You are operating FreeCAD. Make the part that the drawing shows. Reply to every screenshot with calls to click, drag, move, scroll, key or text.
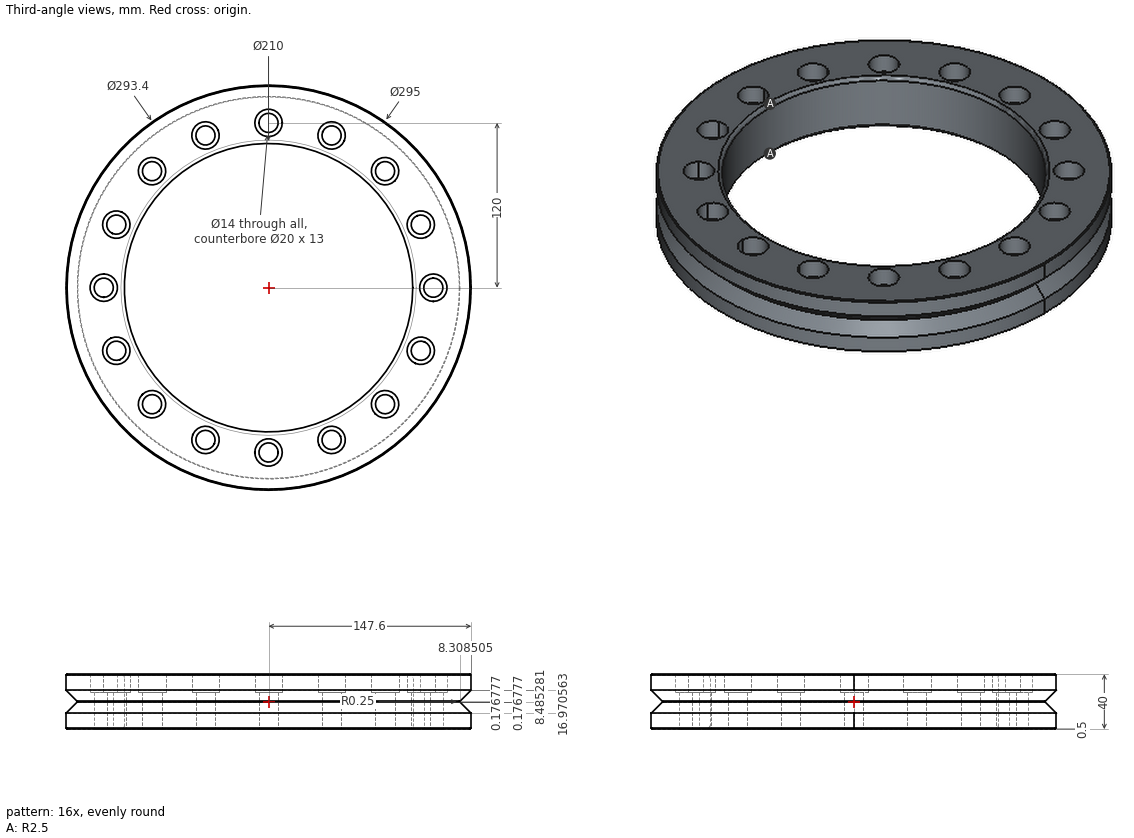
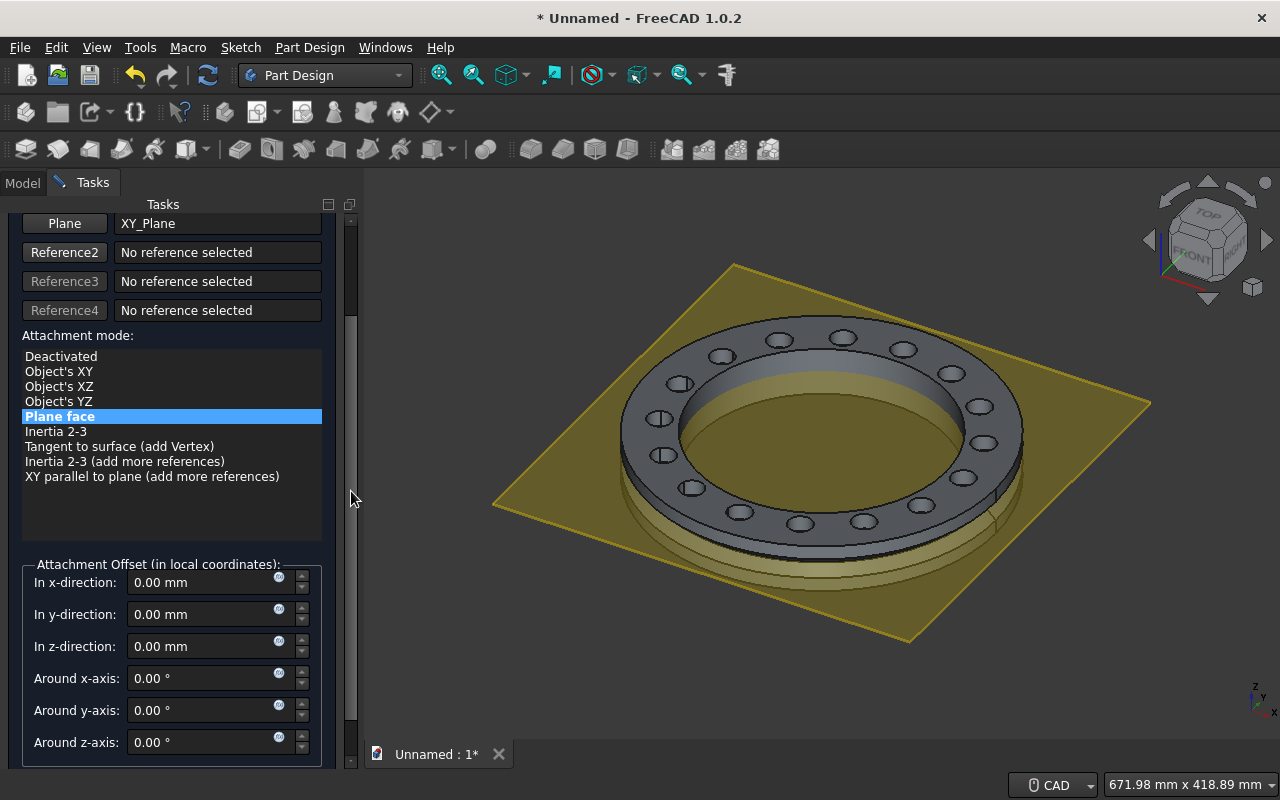
triple_click(210, 646)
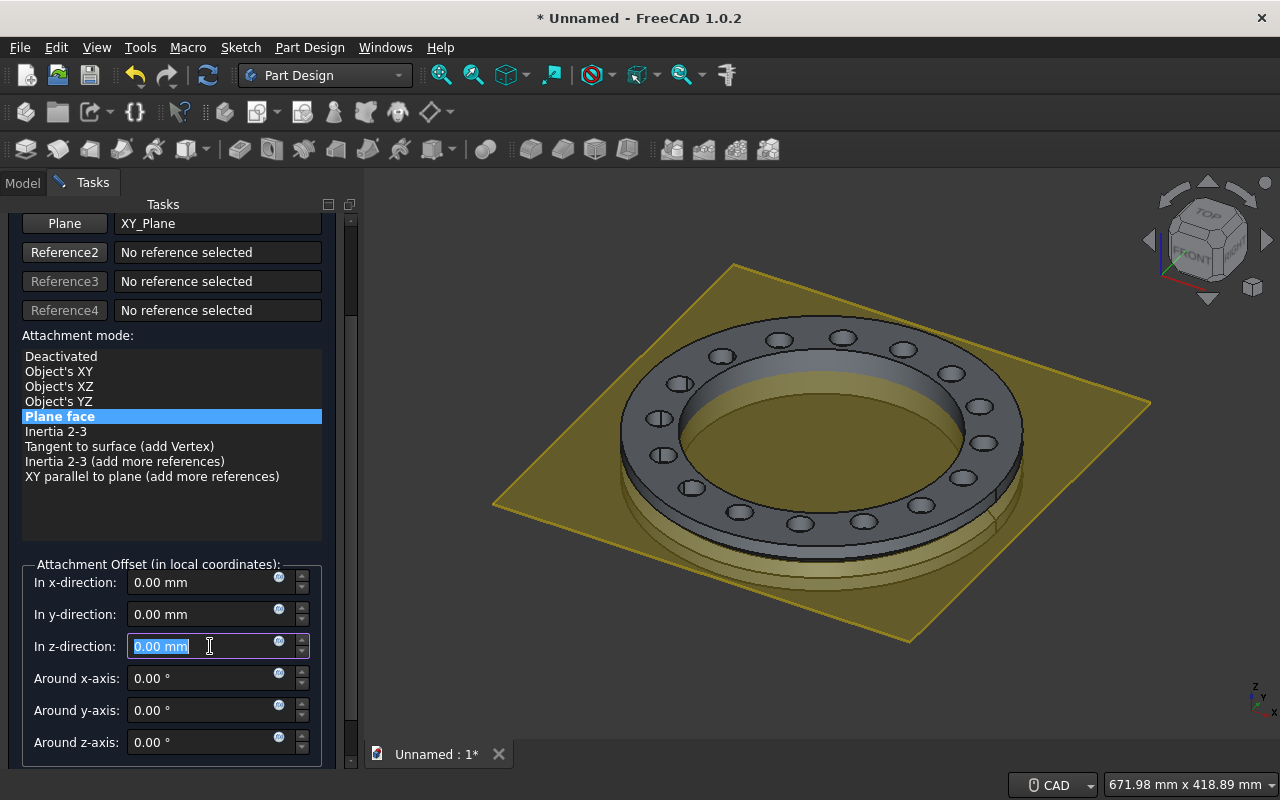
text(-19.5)
key(Tab)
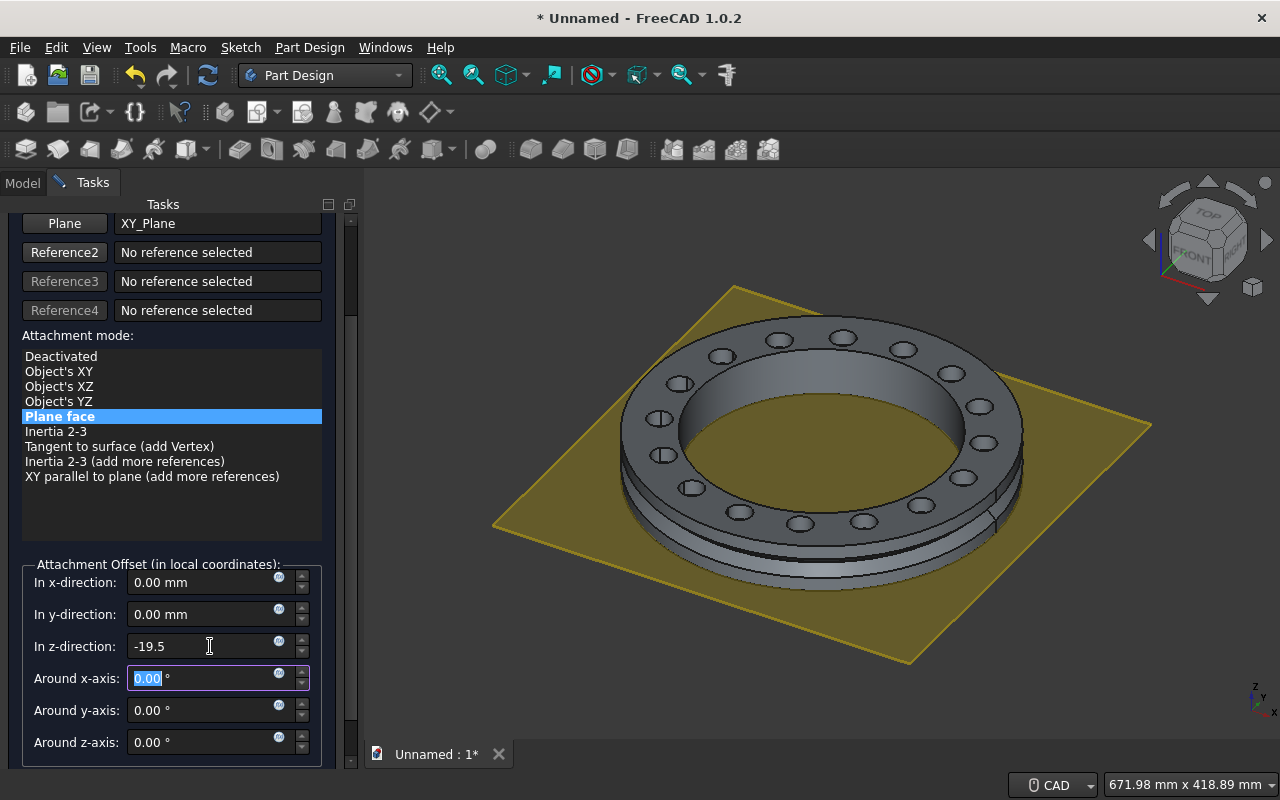
scroll(351, 491, up, 3)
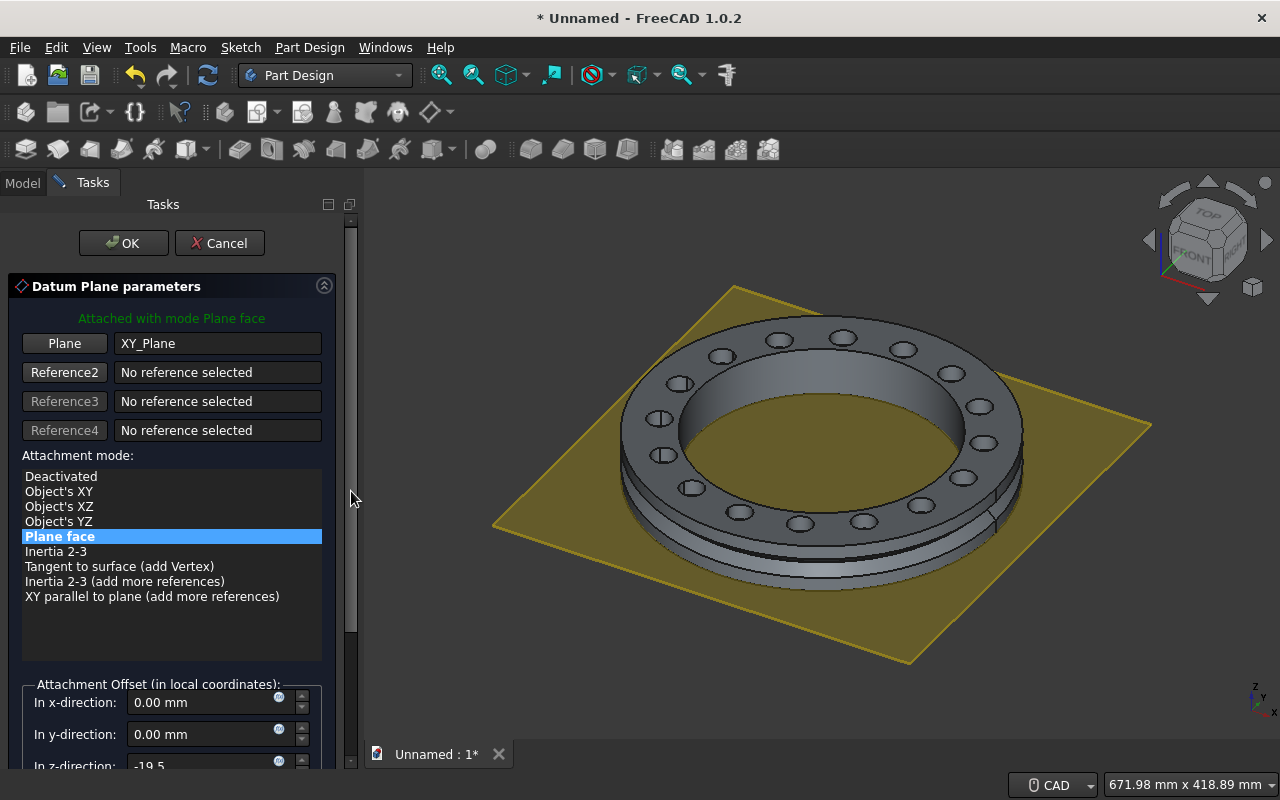
click(124, 243)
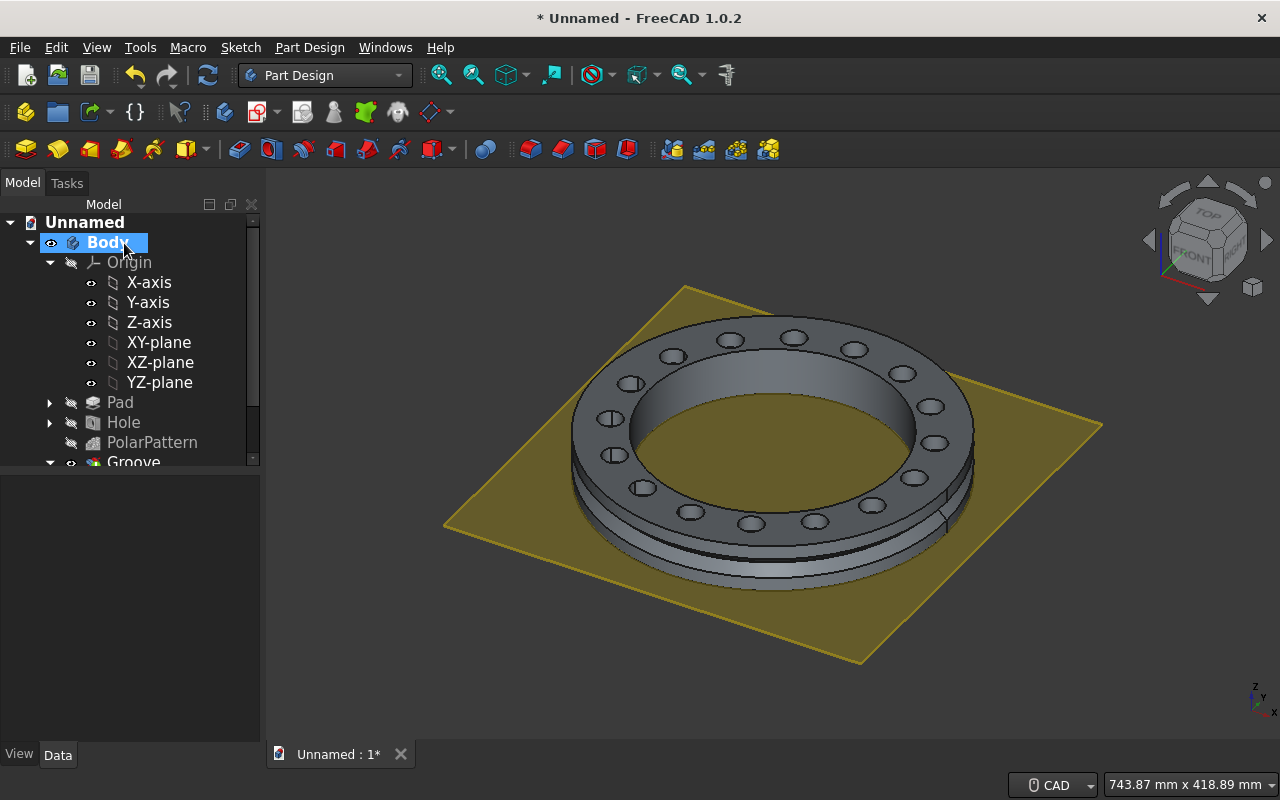
scroll(100, 338, down, 3)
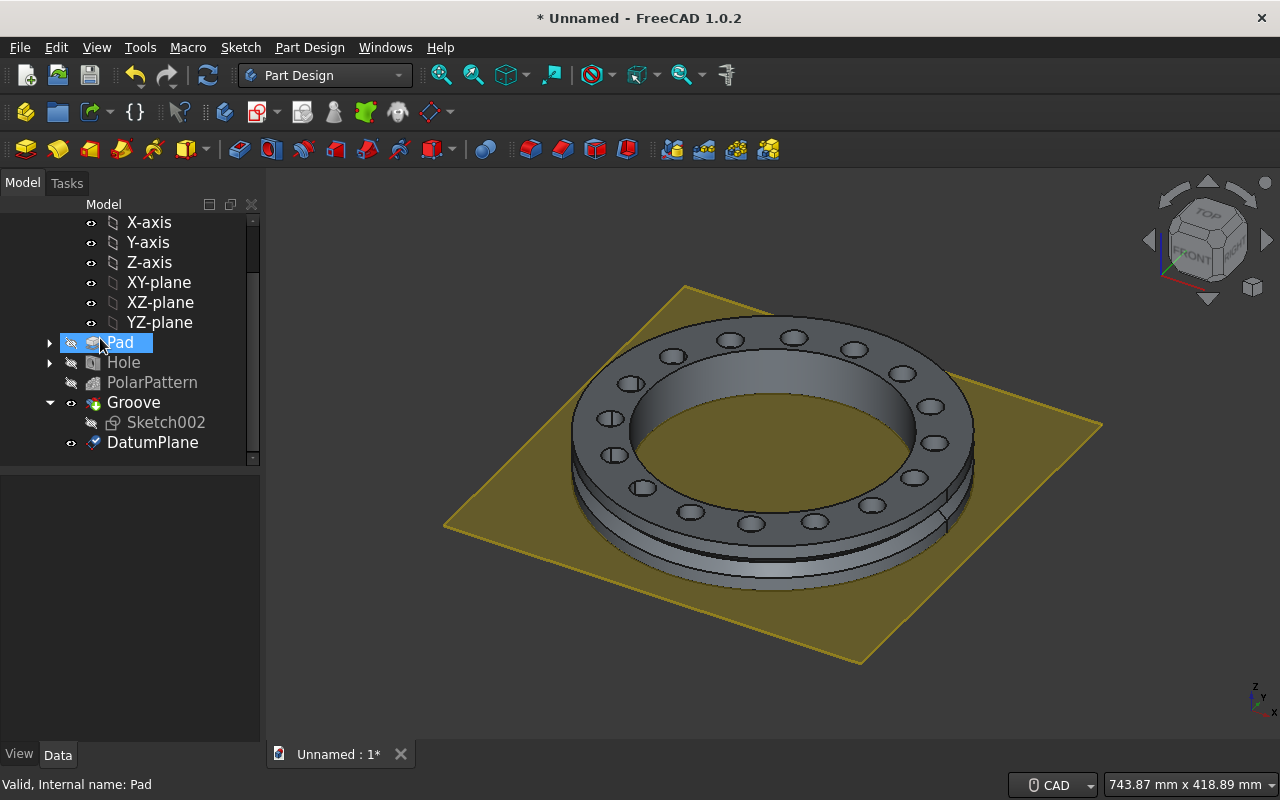
click(116, 443)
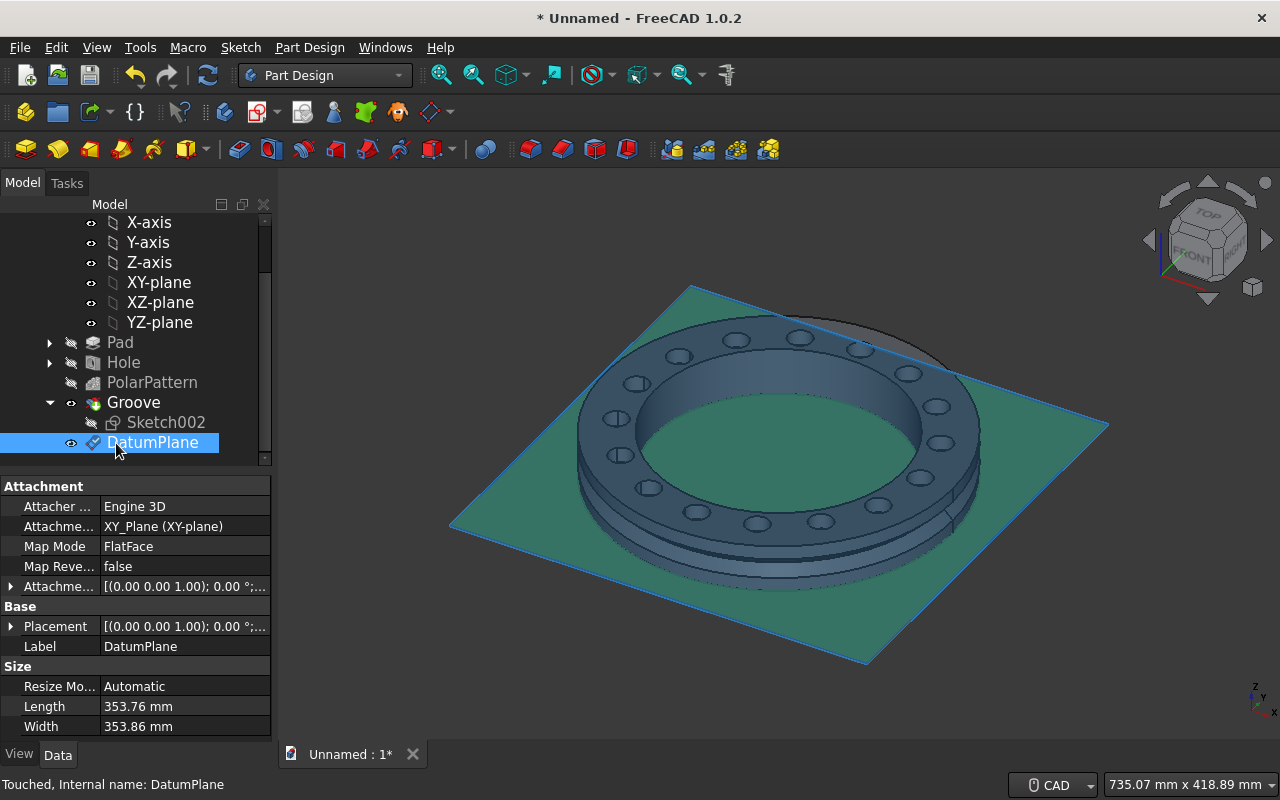
click(258, 112)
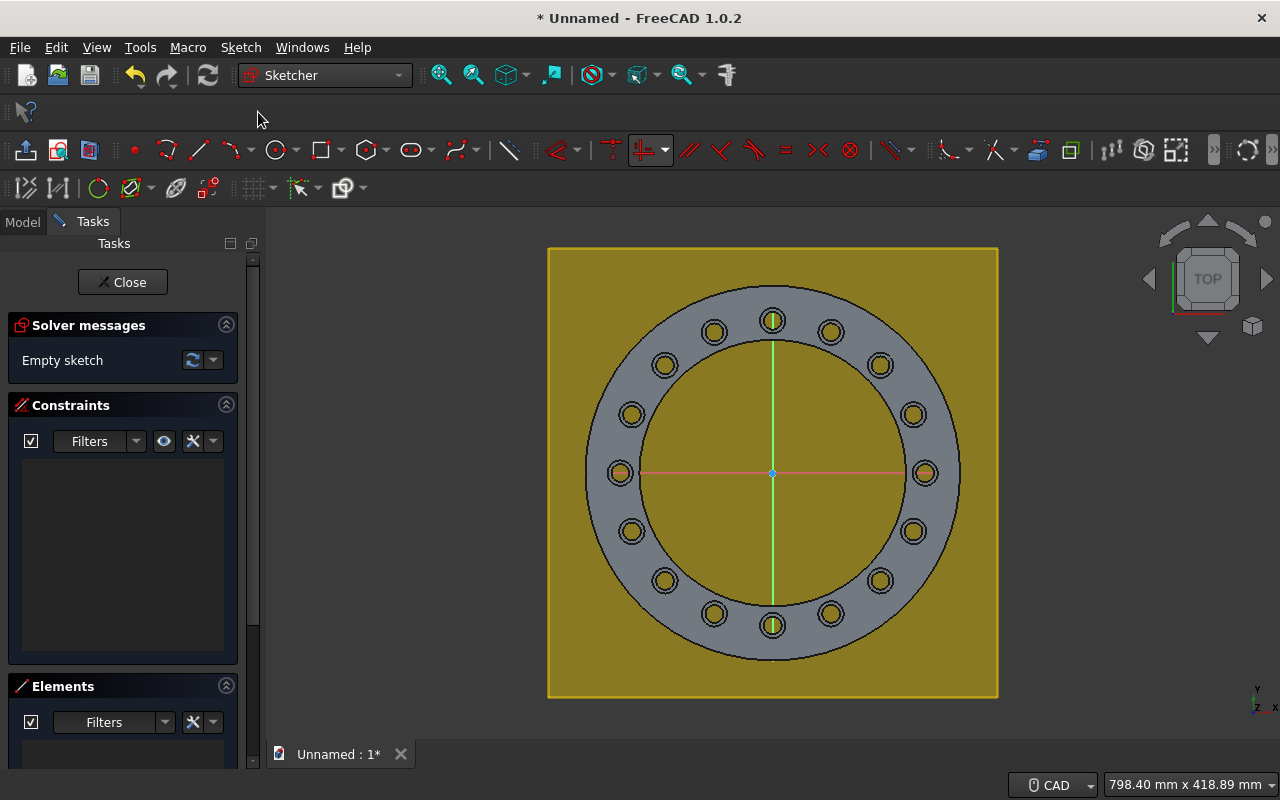
click(90, 150)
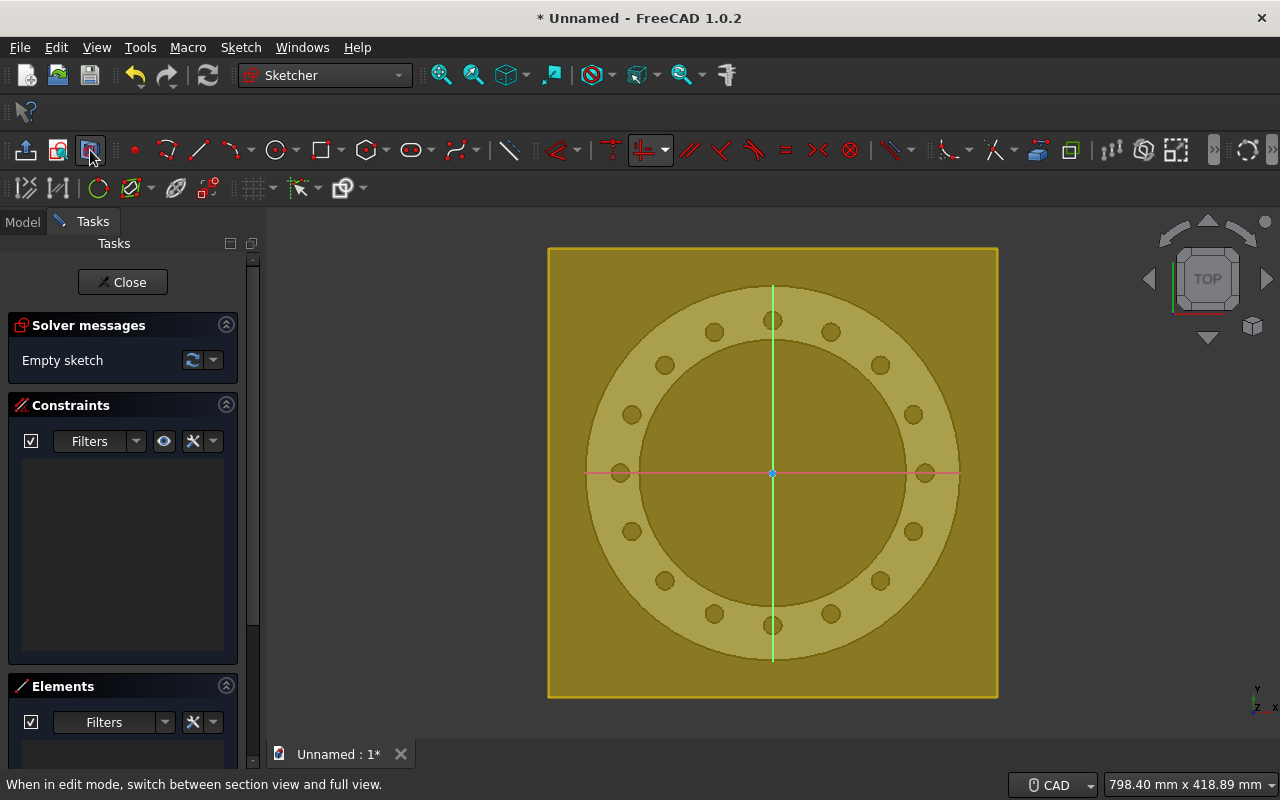
click(276, 150)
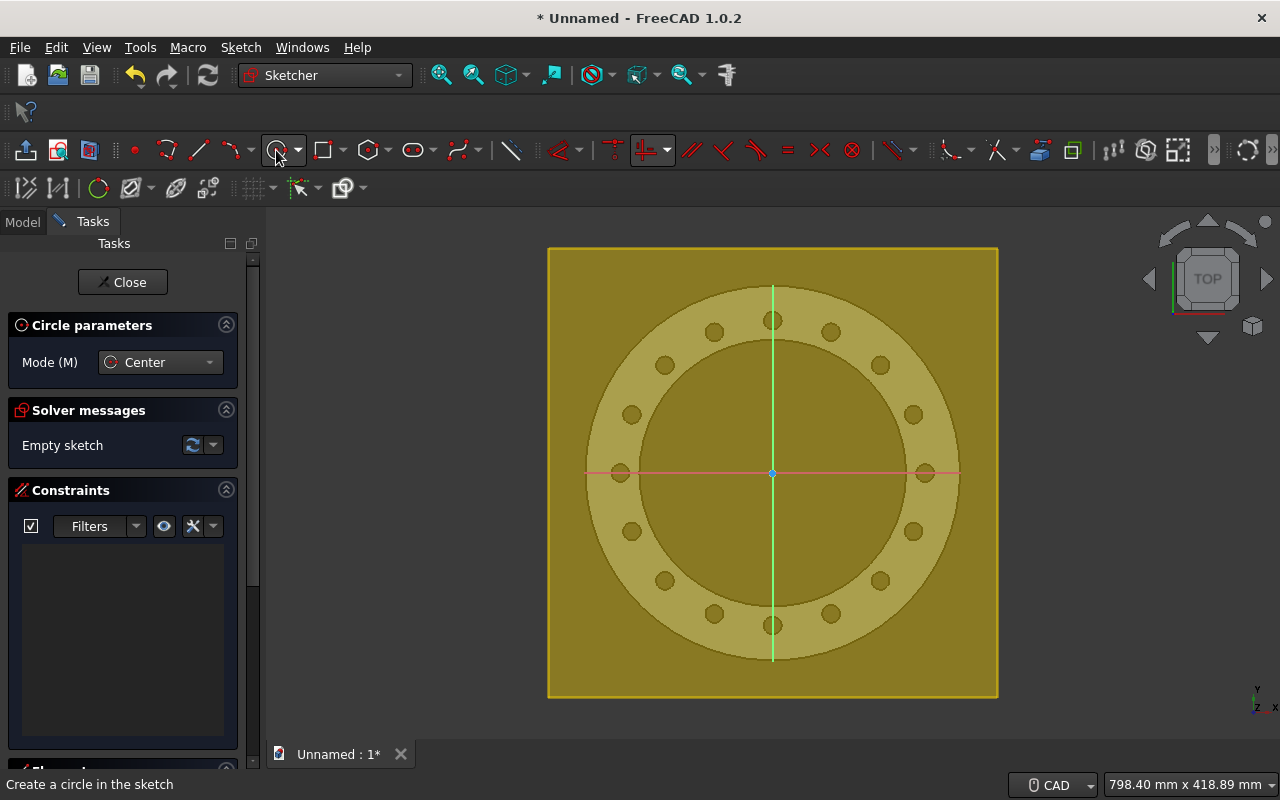
click(773, 473)
move(905, 341)